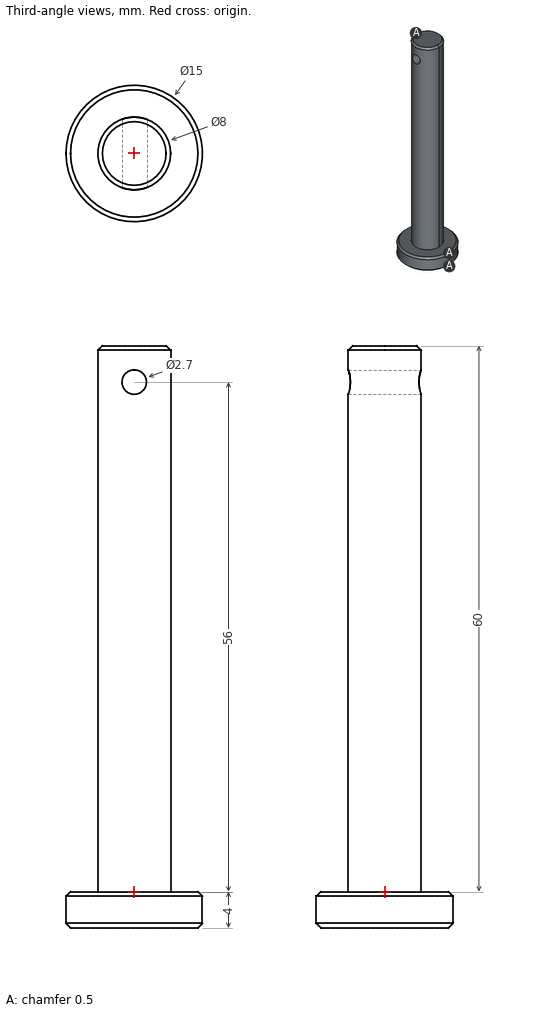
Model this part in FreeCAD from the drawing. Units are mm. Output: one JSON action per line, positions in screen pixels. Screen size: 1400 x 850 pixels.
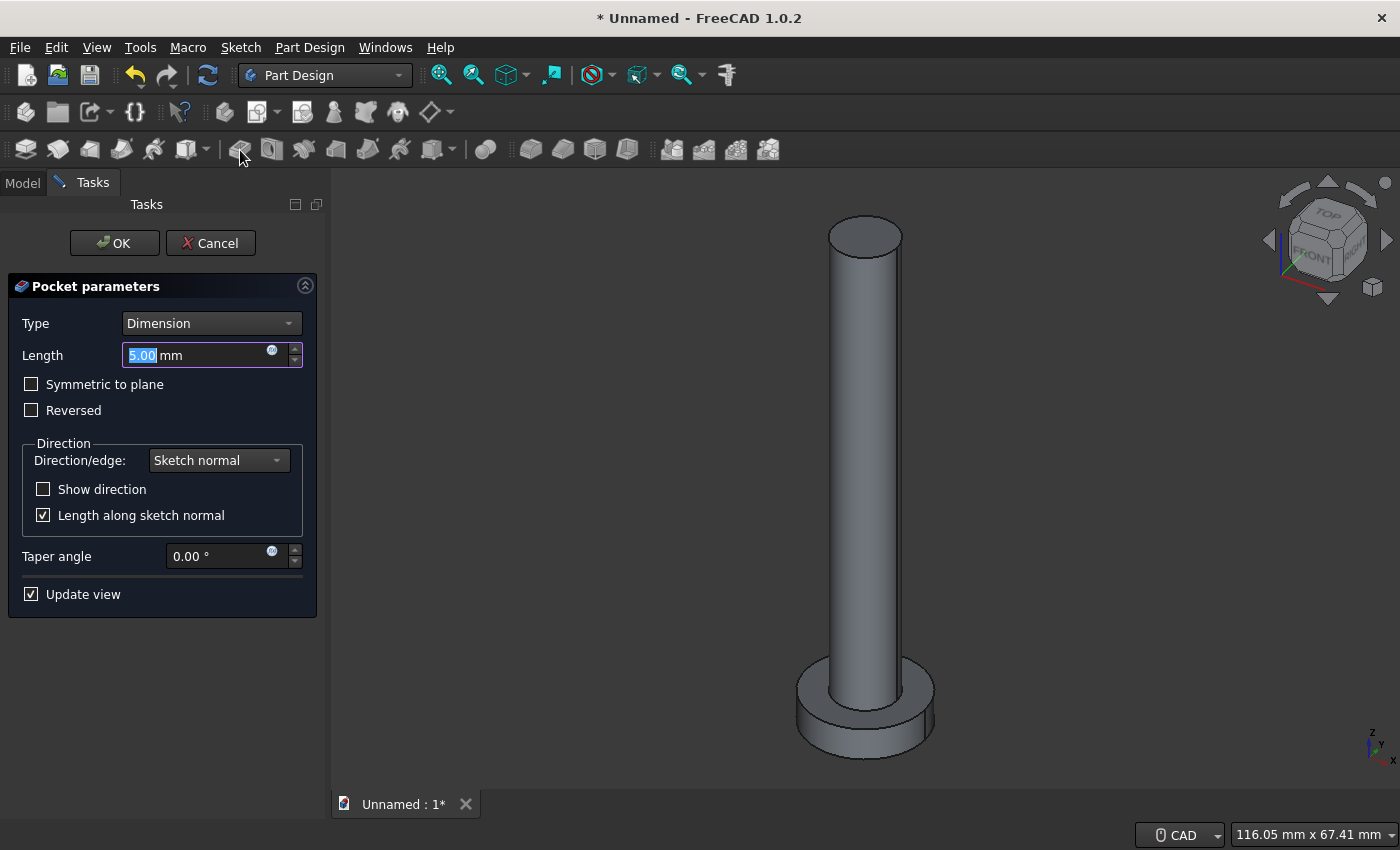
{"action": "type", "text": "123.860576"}
{"action": "key", "text": "Tab"}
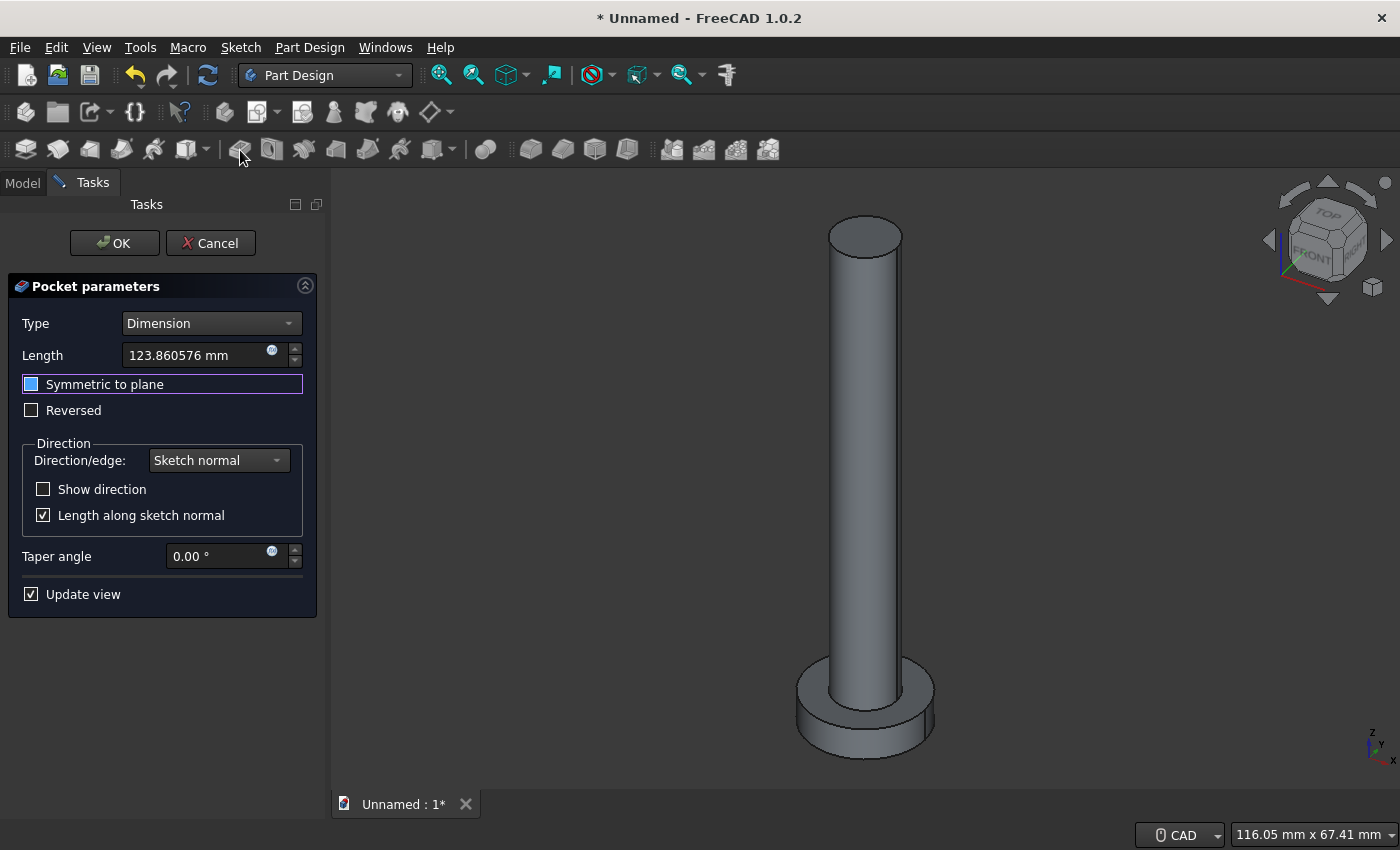
{"action": "left_click", "coordinate": [30, 384]}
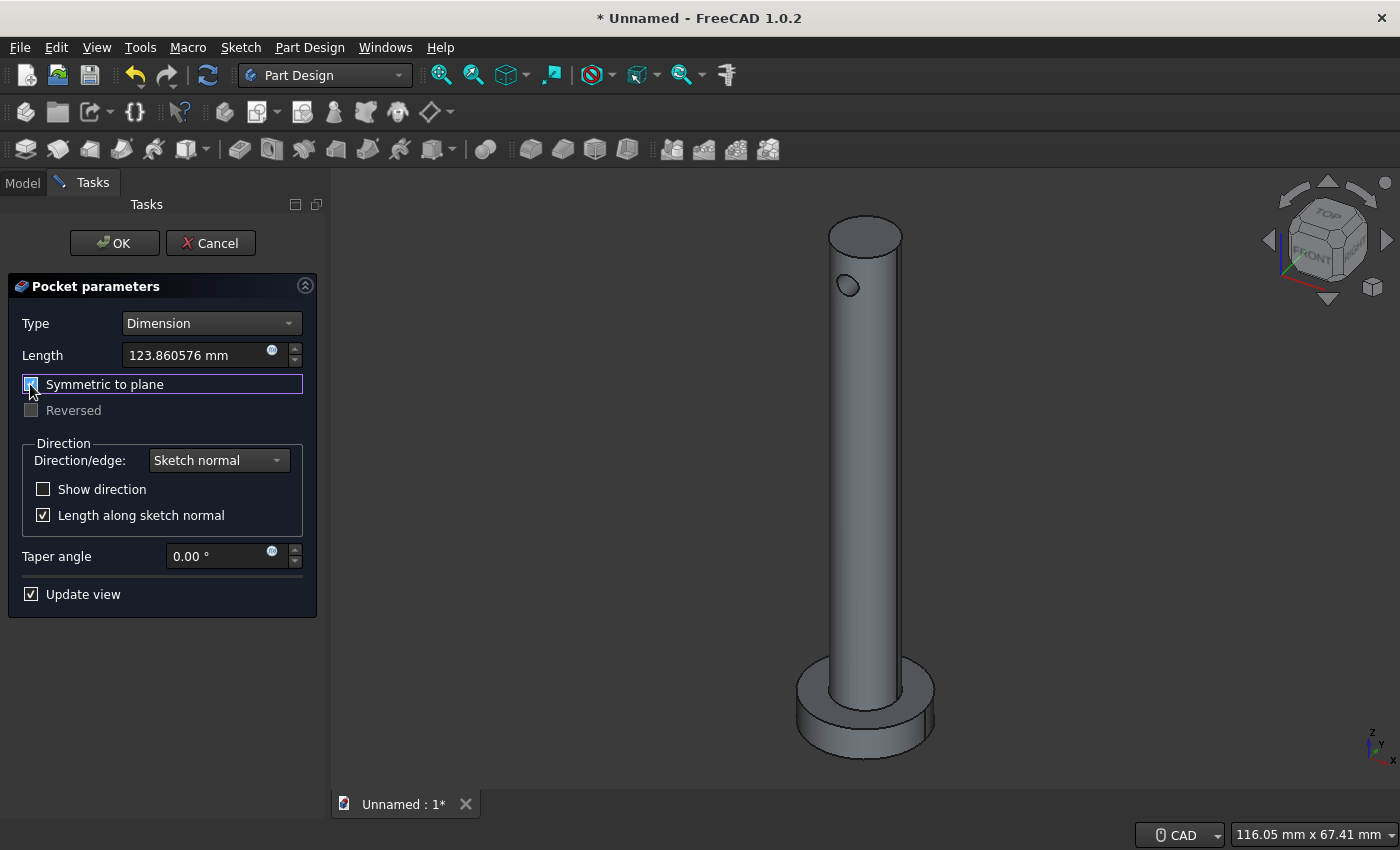
{"action": "left_click", "coordinate": [115, 243]}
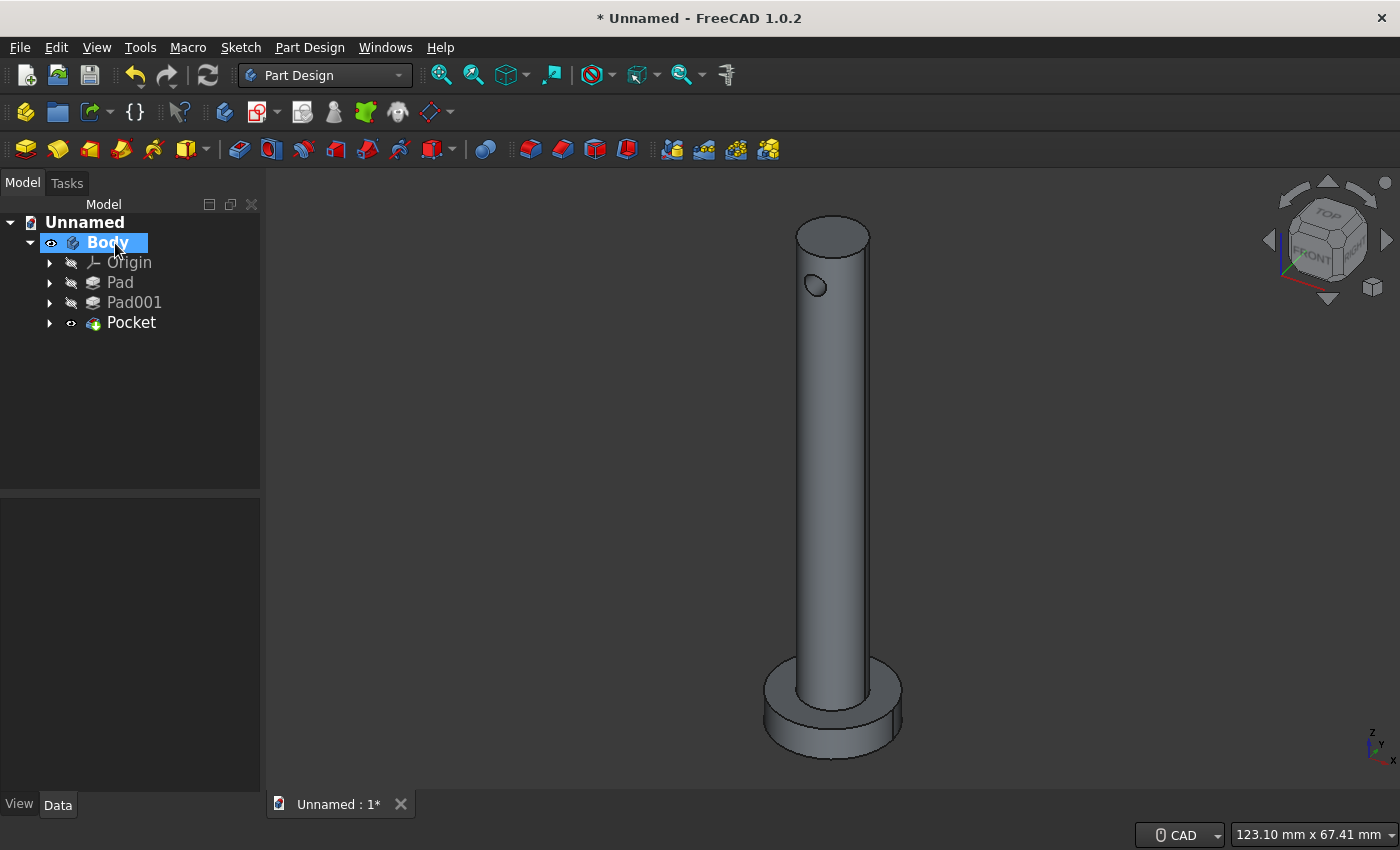
{"action": "left_click", "coordinate": [796, 238]}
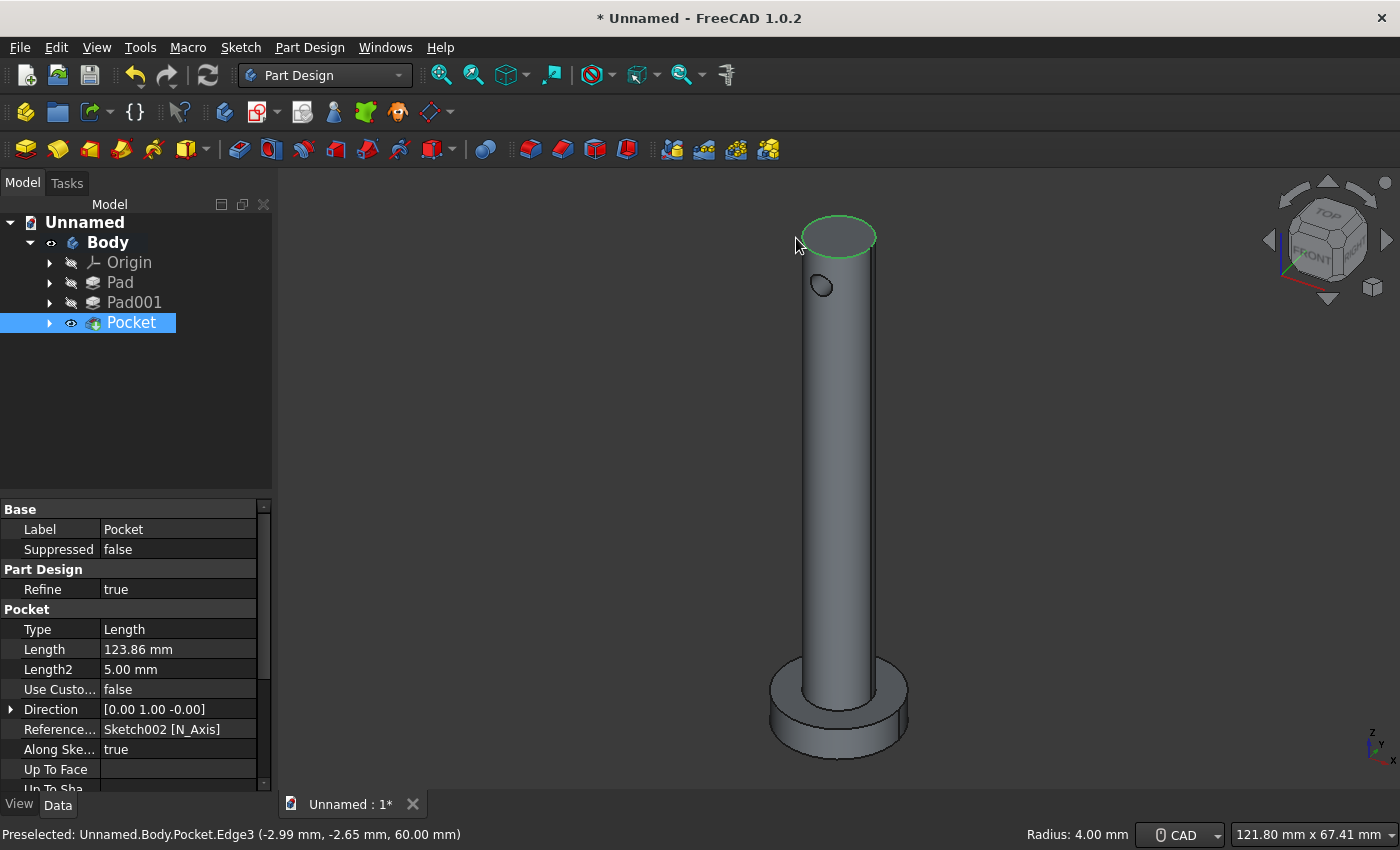
{"action": "left_click", "coordinate": [770, 693], "text": "ctrl"}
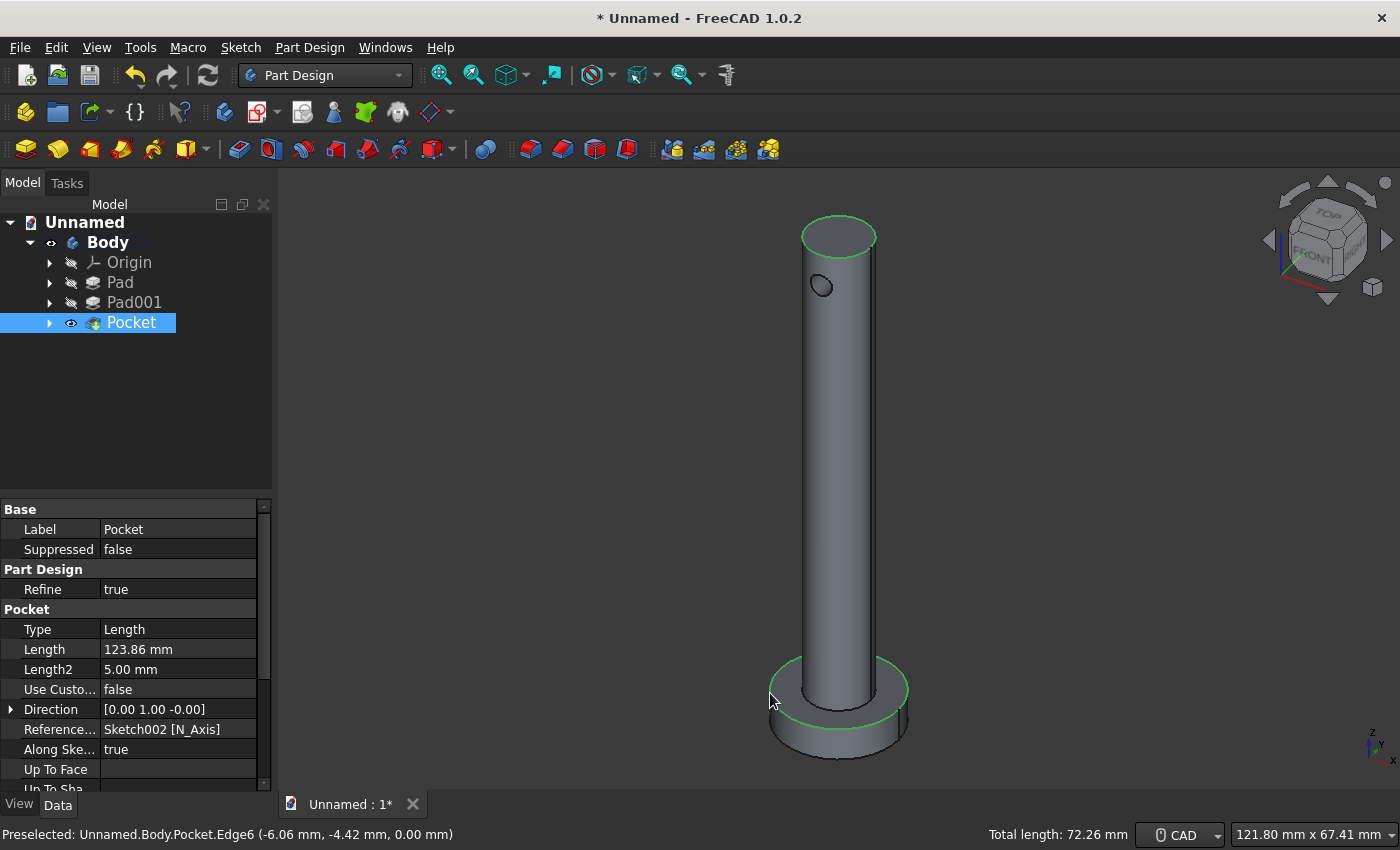
{"action": "key", "text": "0"}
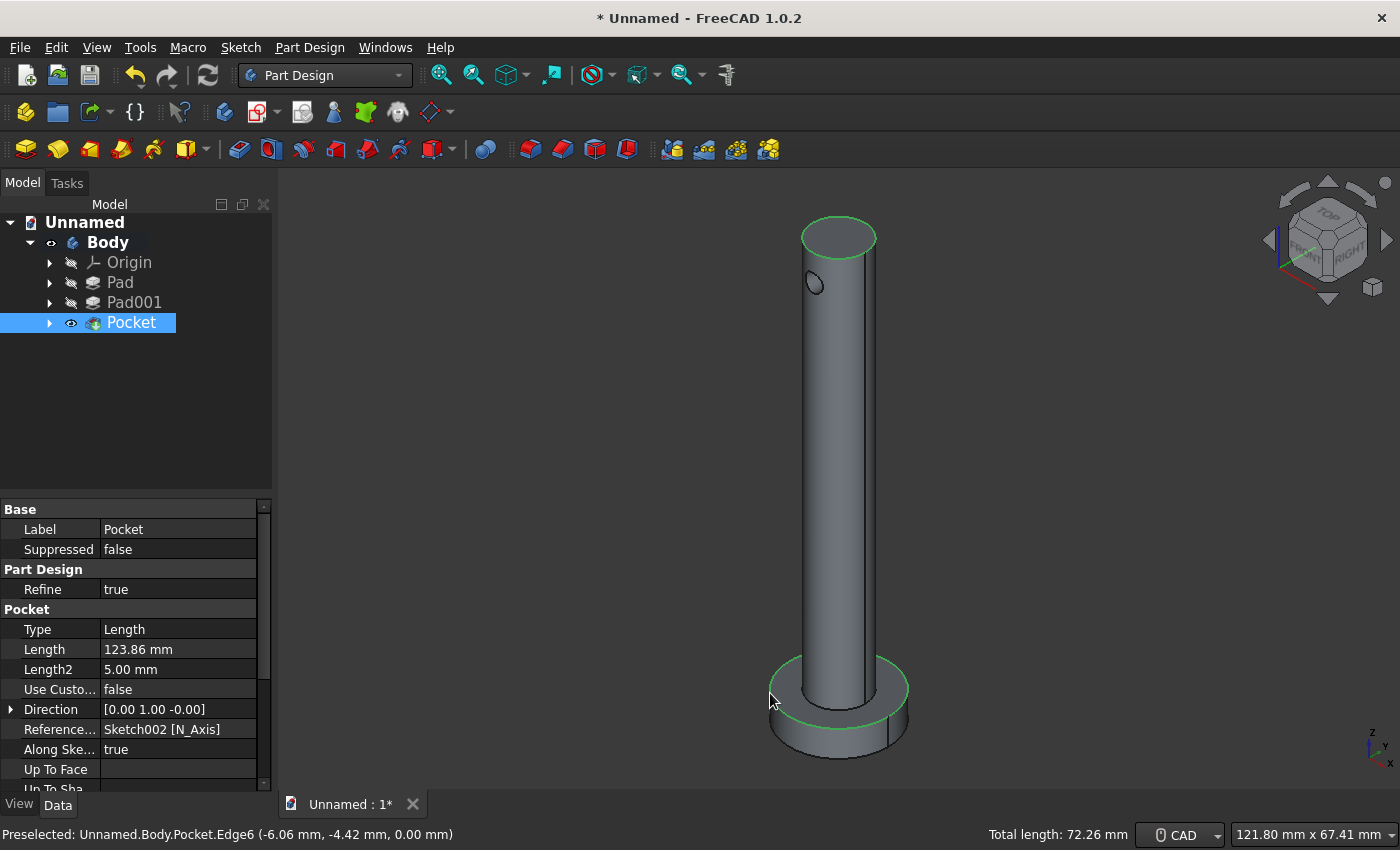
{"action": "key", "text": "2"}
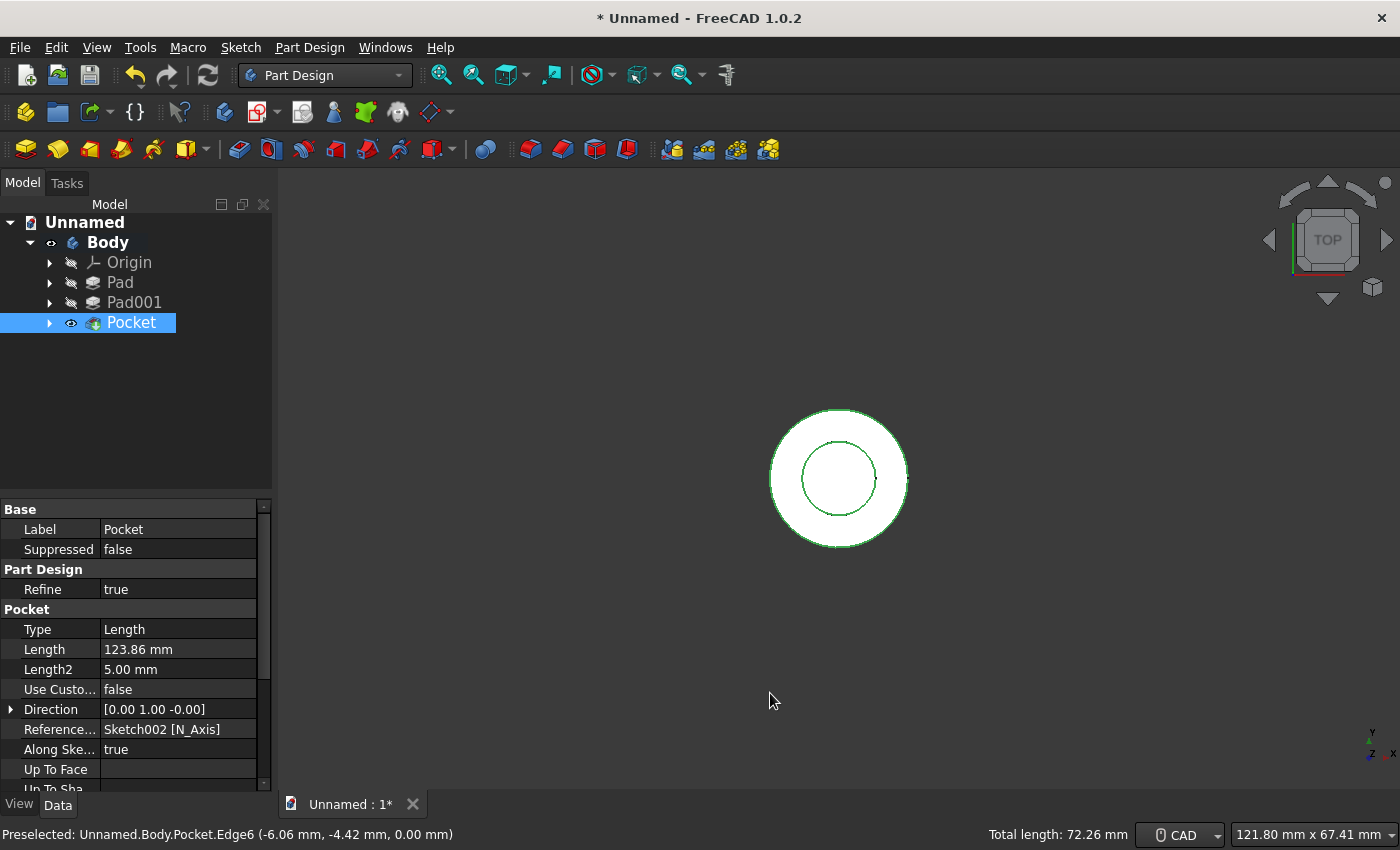
{"action": "left_click", "coordinate": [442, 76]}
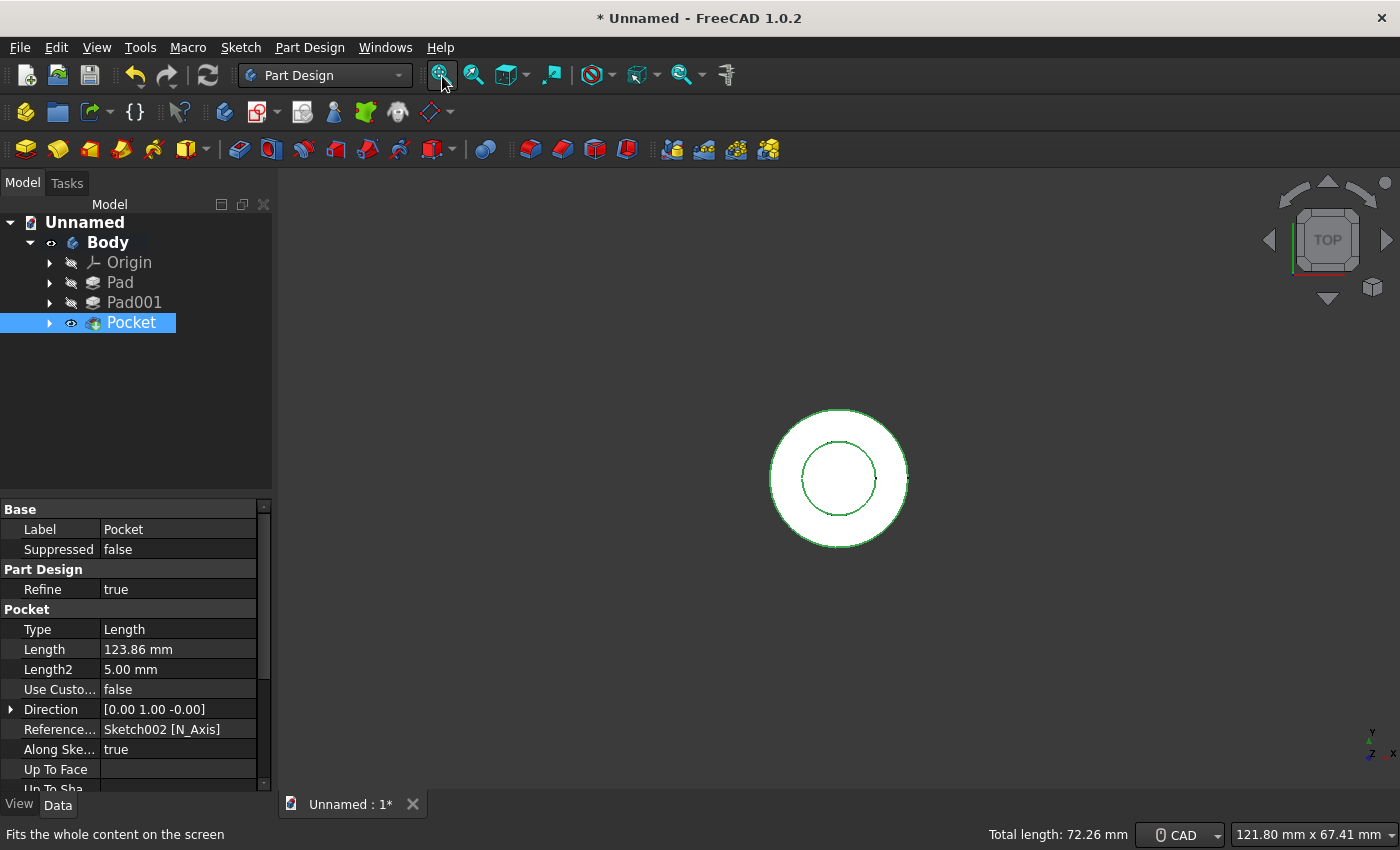
{"action": "key", "text": "1"}